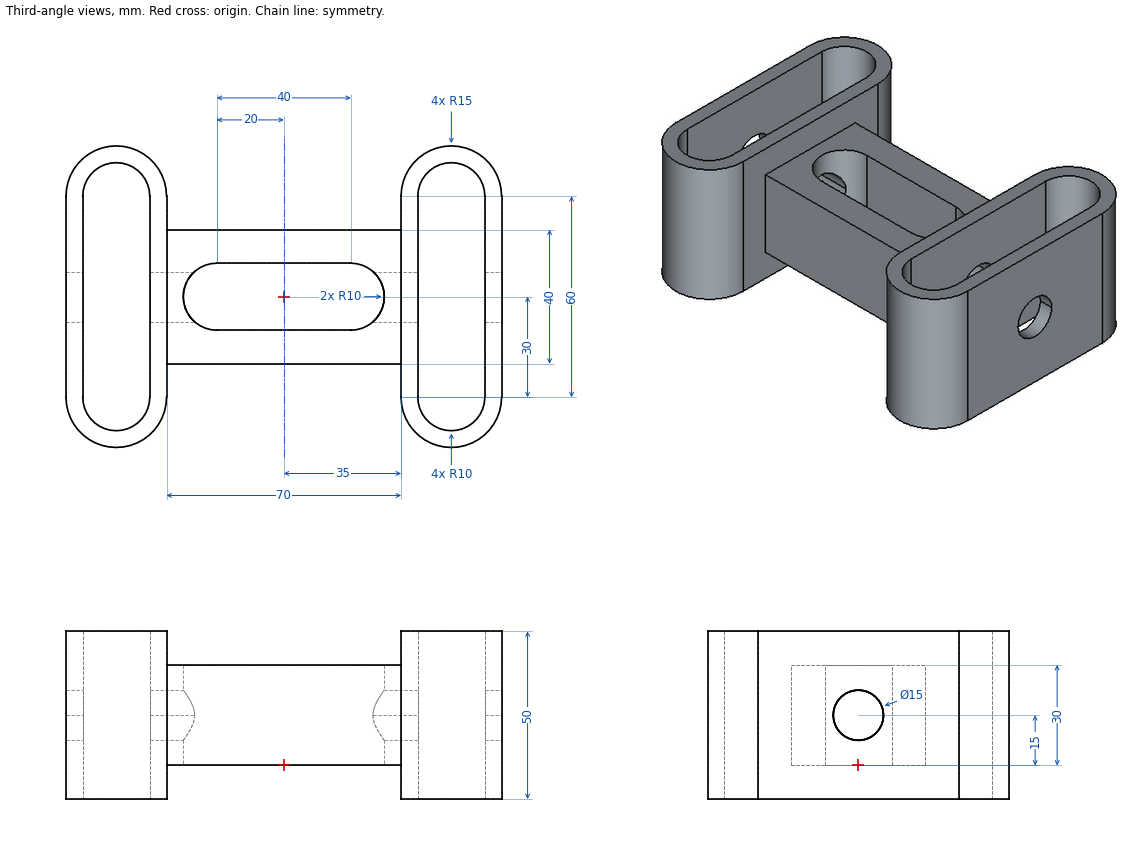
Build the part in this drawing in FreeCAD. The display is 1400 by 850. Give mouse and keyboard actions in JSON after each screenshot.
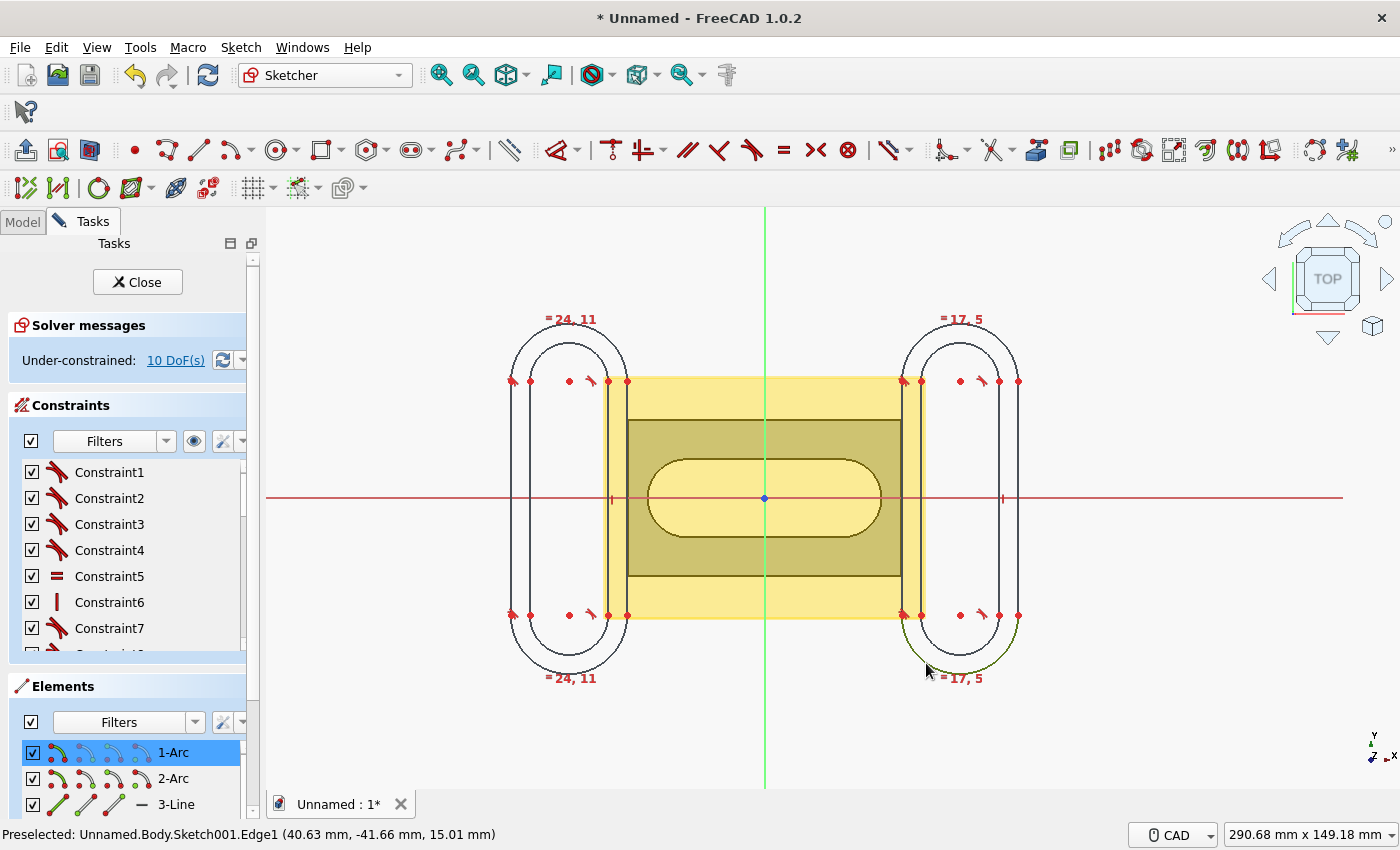
{"action": "left_click", "coordinate": [535, 663]}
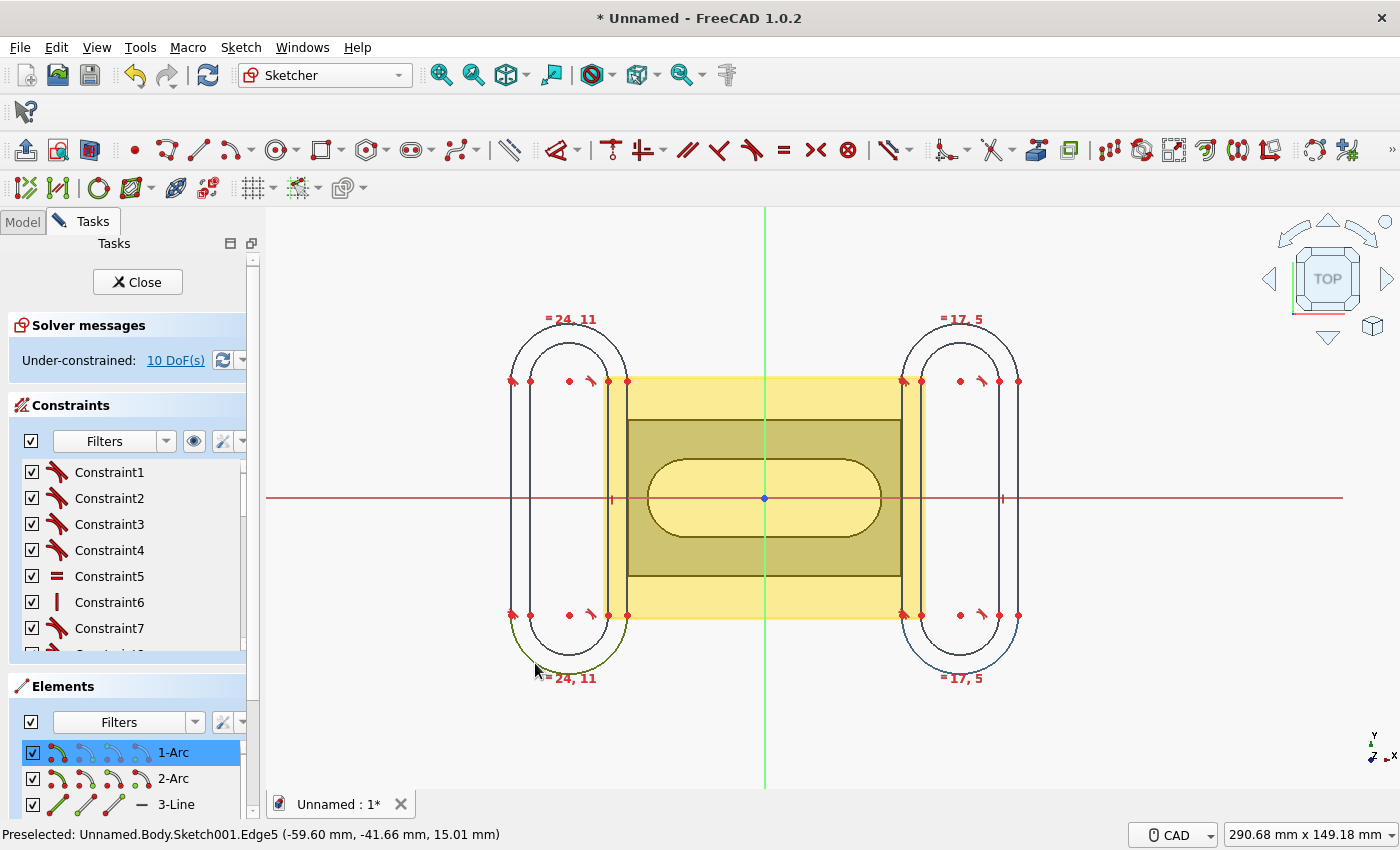
{"action": "key", "text": "e"}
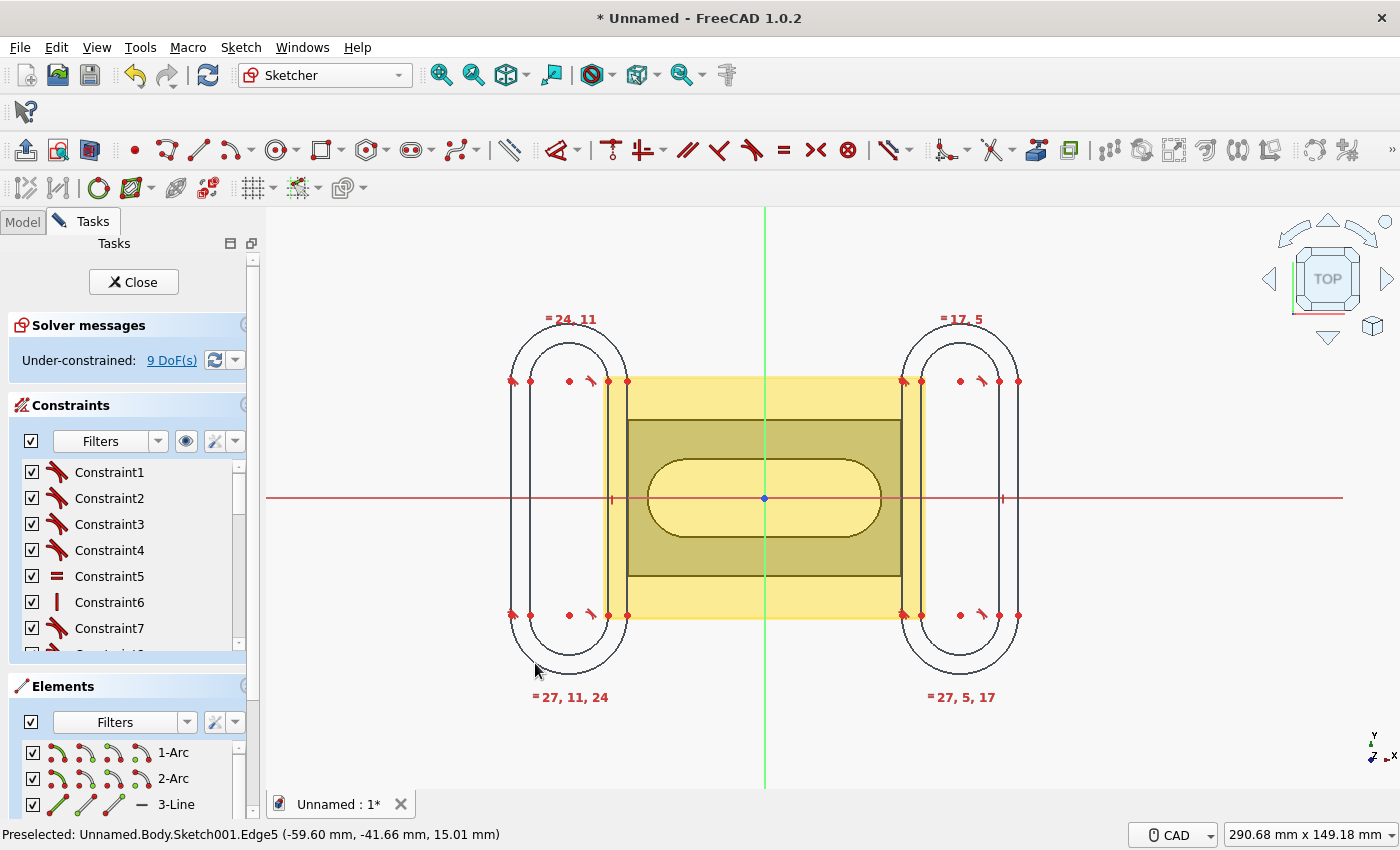
{"action": "left_click", "coordinate": [937, 648]}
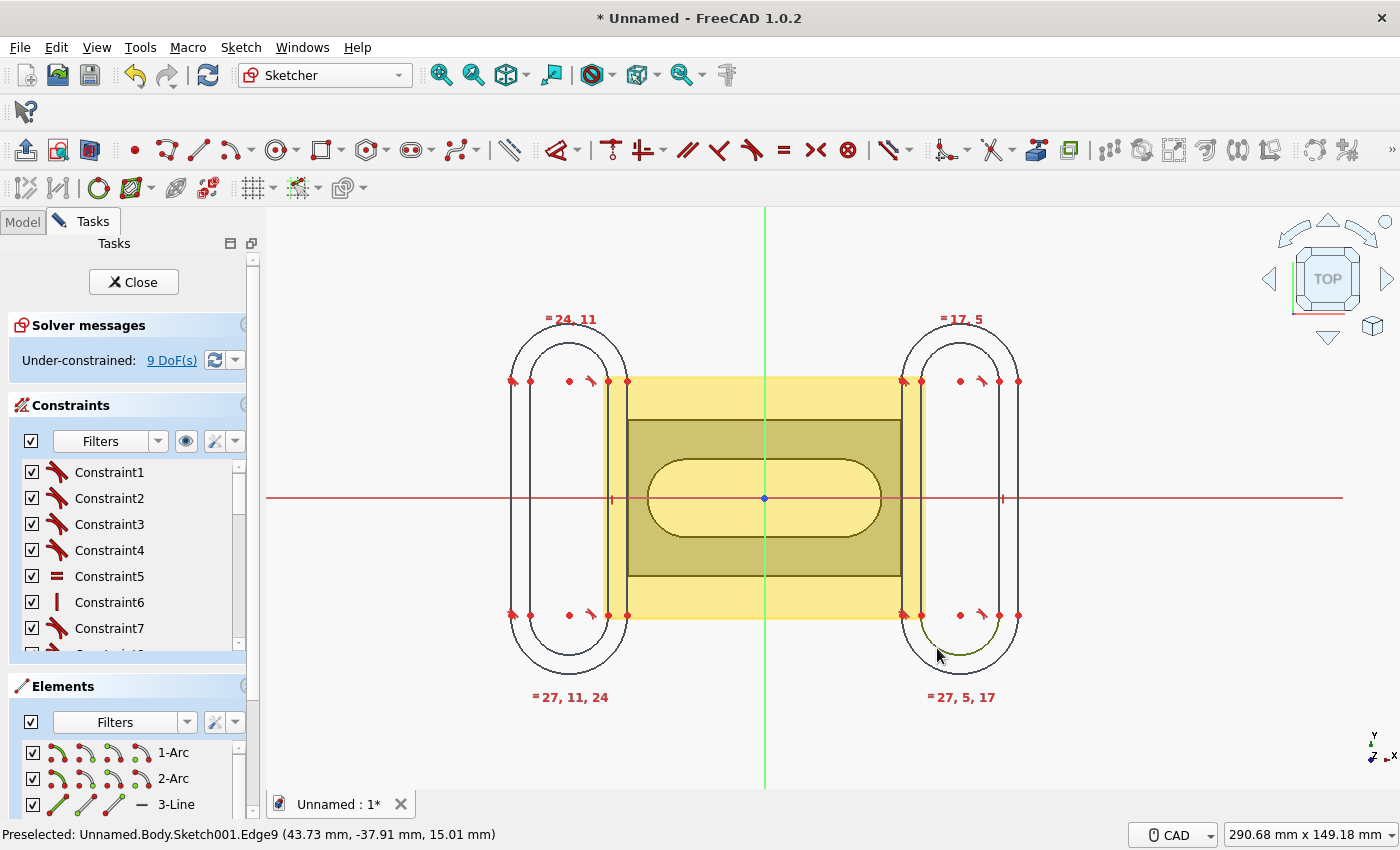
{"action": "left_click", "coordinate": [546, 648]}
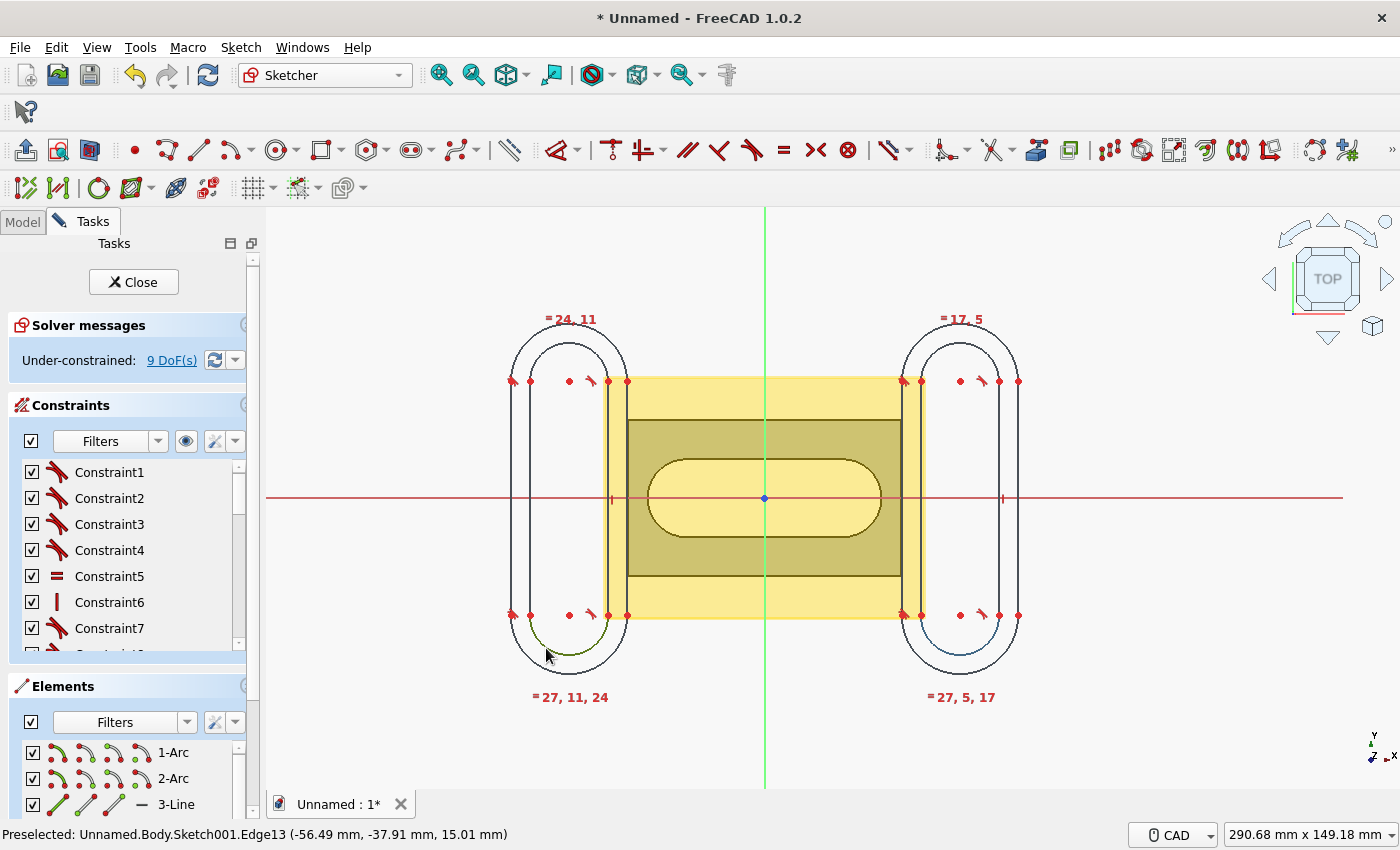
{"action": "key", "text": "e"}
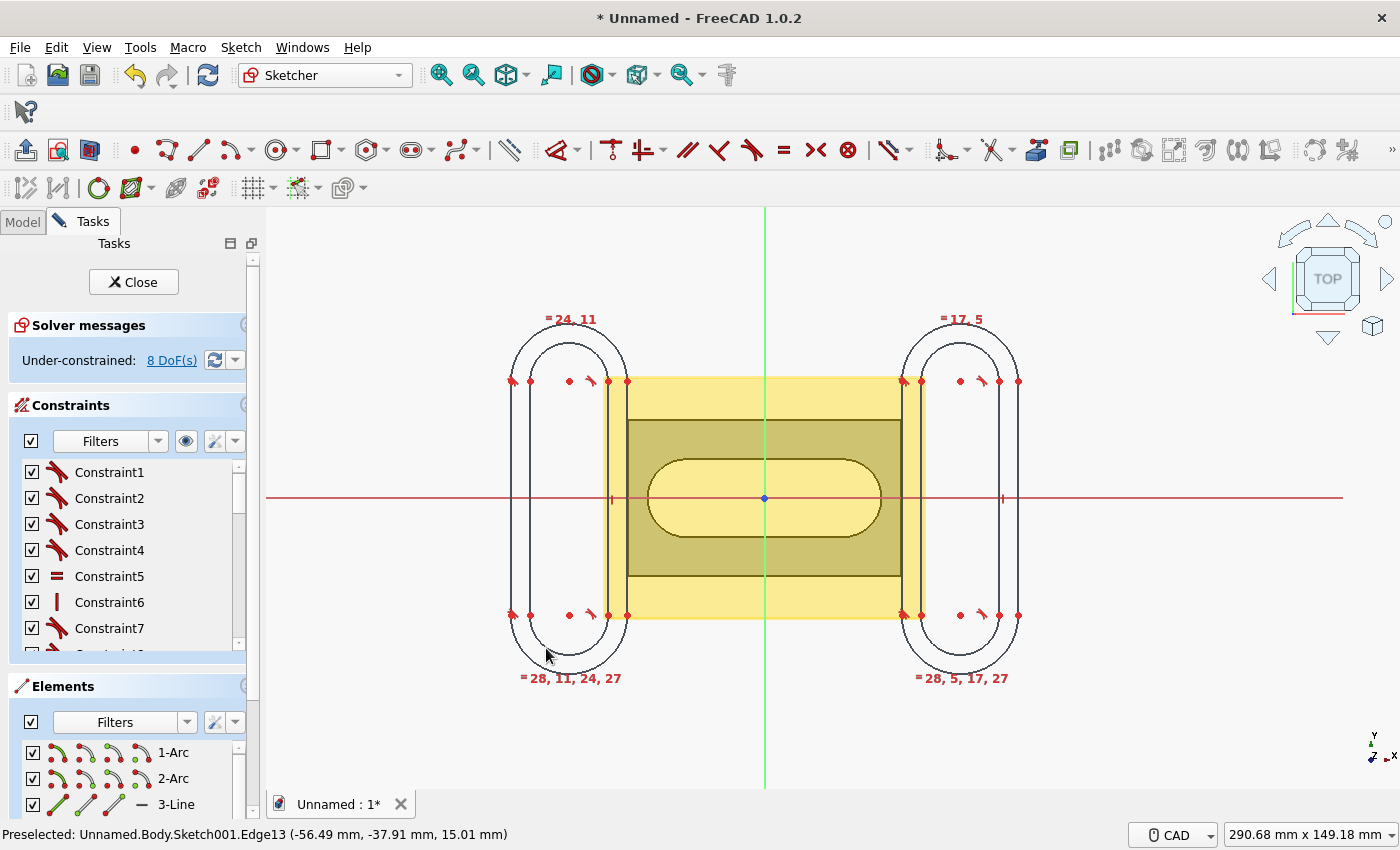
{"action": "left_click", "coordinate": [960, 616]}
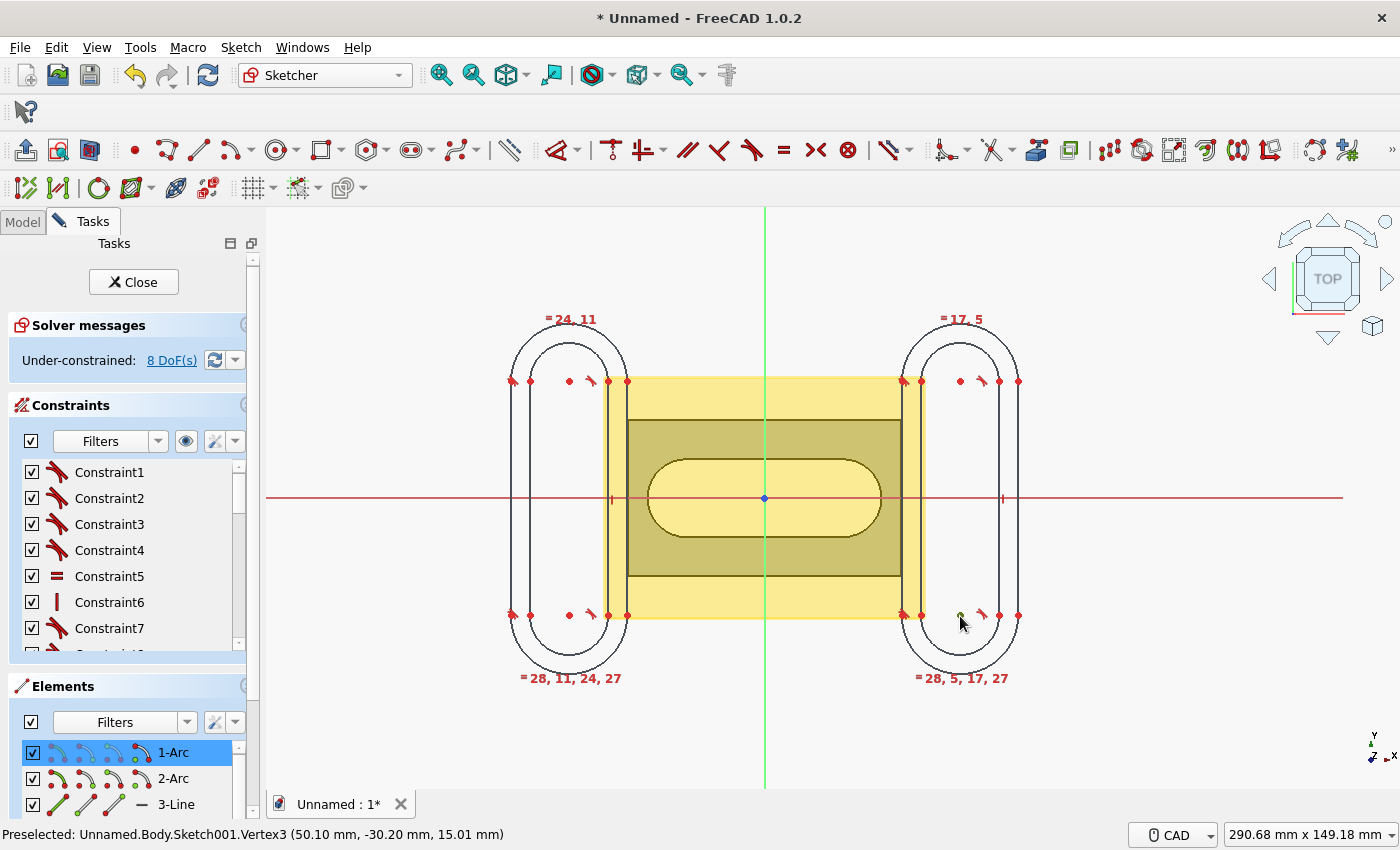
{"action": "left_click", "coordinate": [569, 616]}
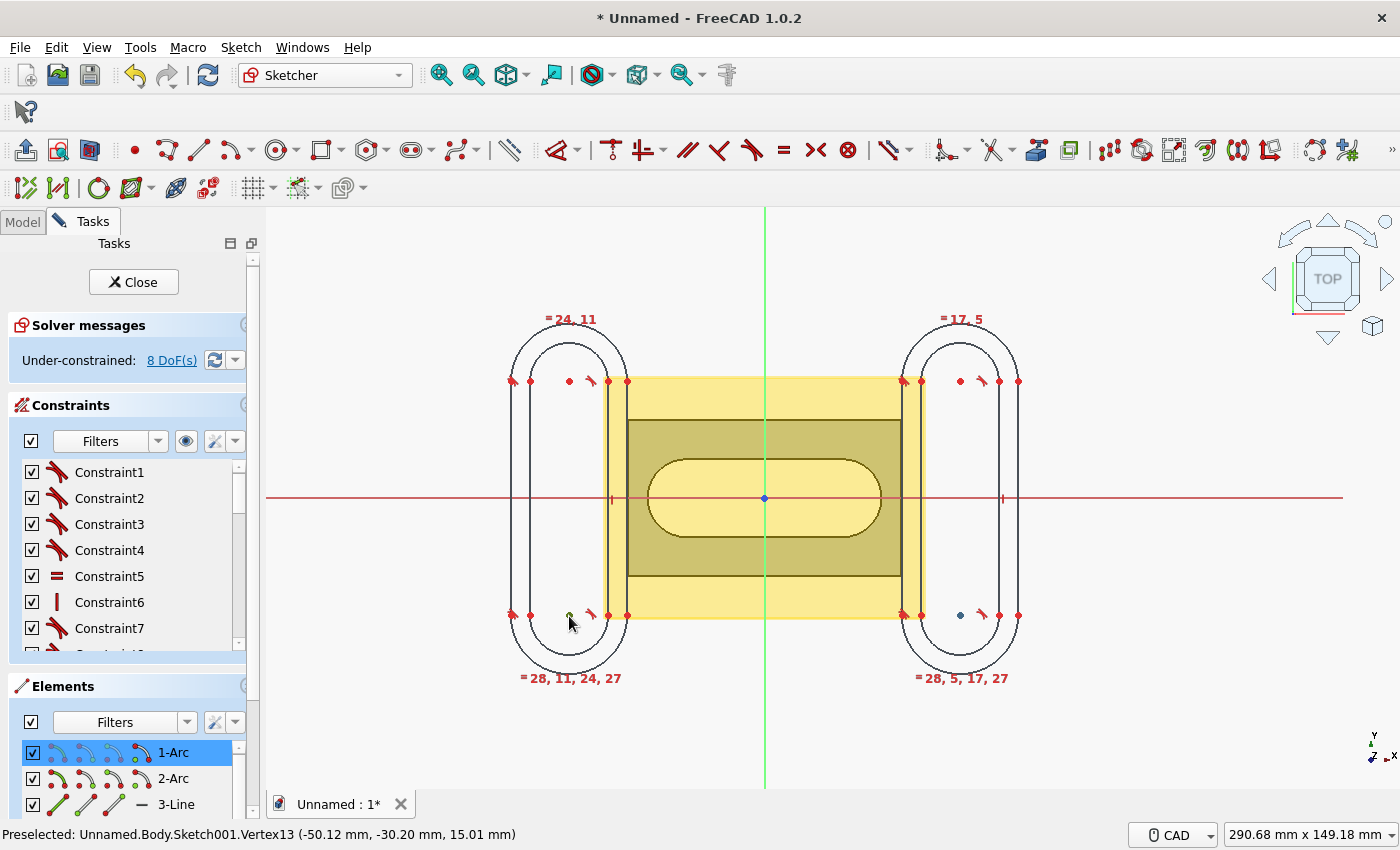
{"action": "left_click", "coordinate": [765, 723]}